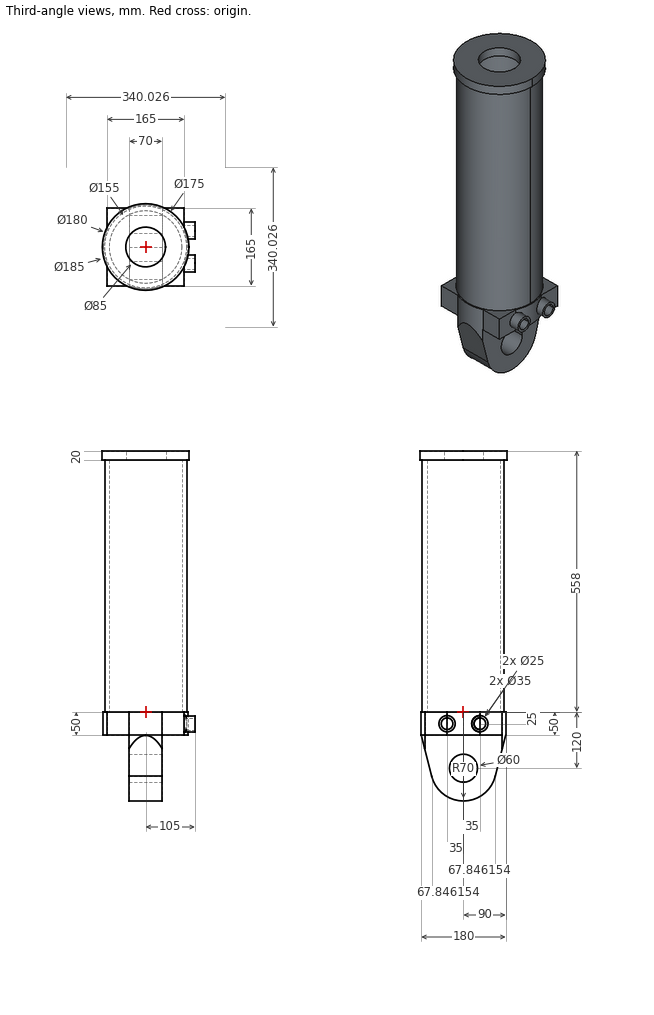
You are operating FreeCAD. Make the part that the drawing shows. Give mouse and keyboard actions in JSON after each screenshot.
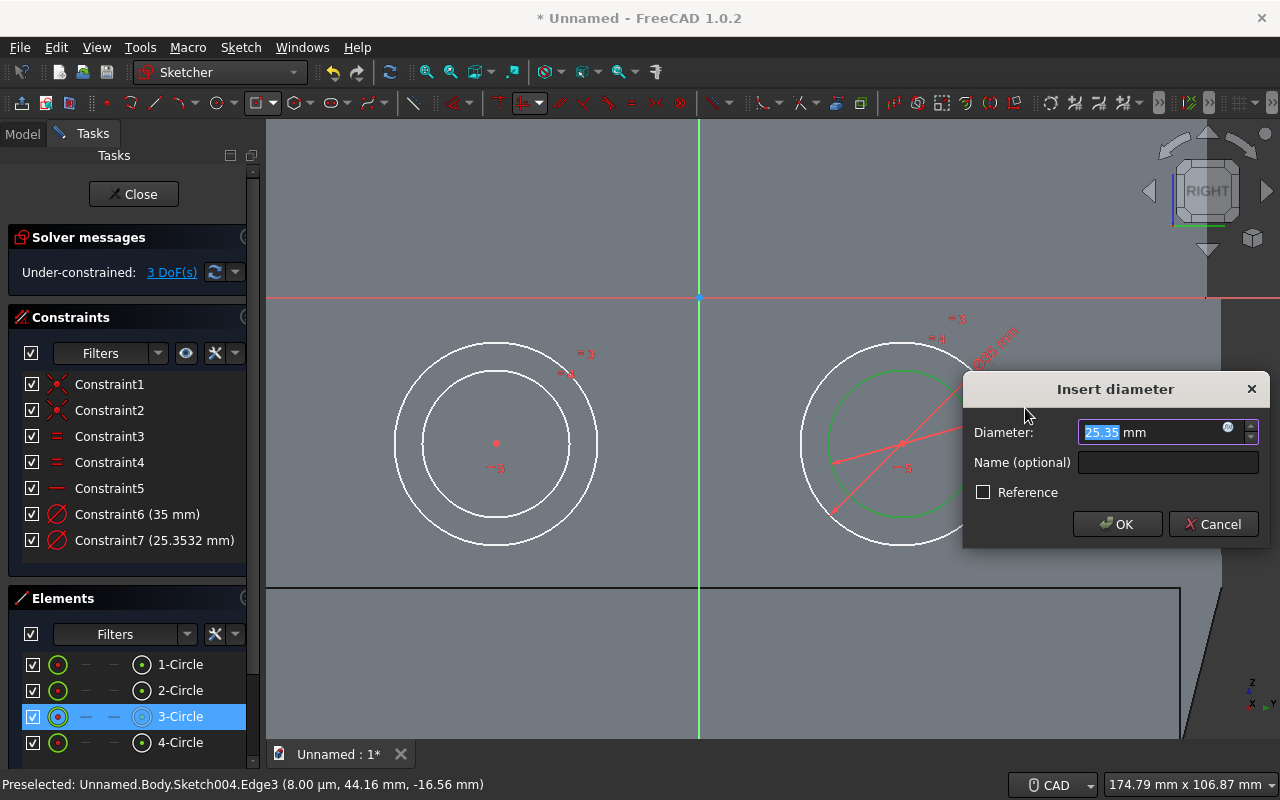
{"action": "type", "text": "25"}
{"action": "key", "text": "Return"}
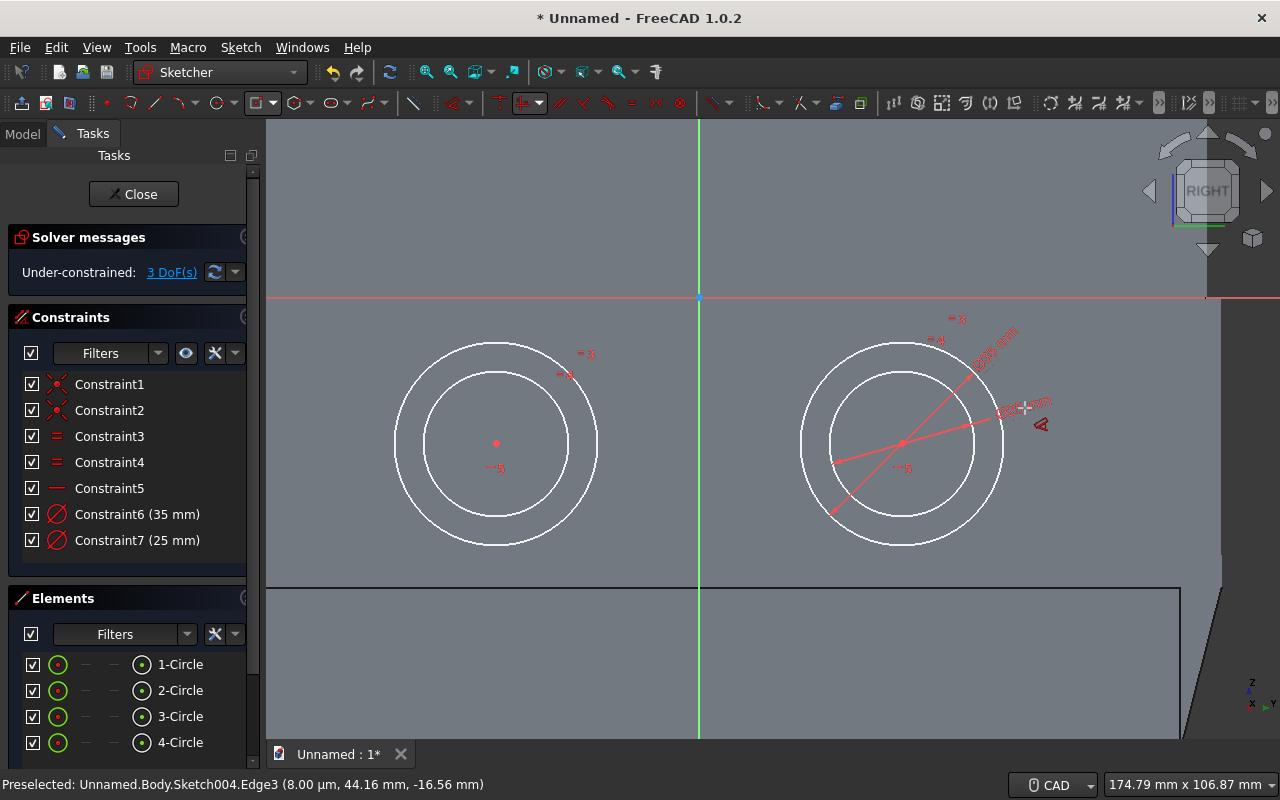
{"action": "left_click", "coordinate": [902, 444]}
{"action": "left_click", "coordinate": [801, 264]}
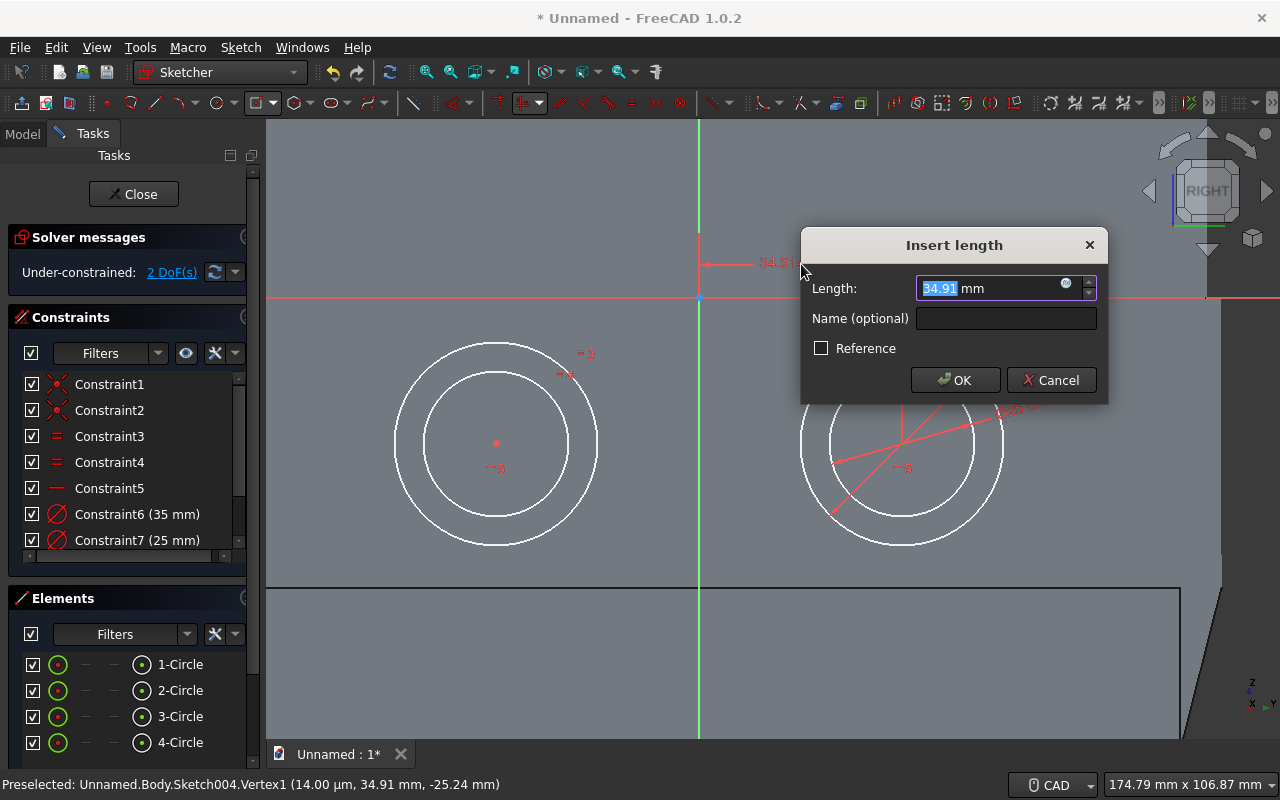
{"action": "type", "text": "35"}
{"action": "key", "text": "Return"}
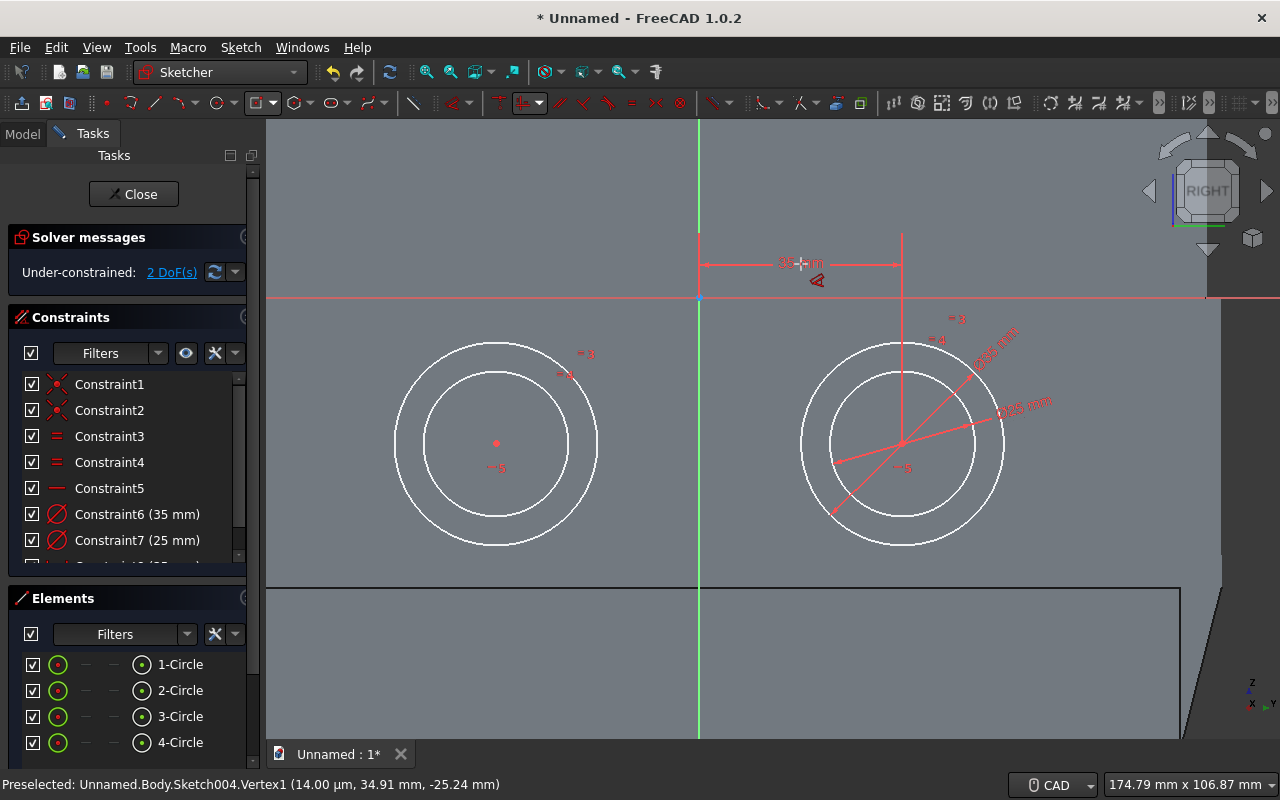
{"action": "left_click", "coordinate": [902, 444]}
{"action": "left_click", "coordinate": [936, 404]}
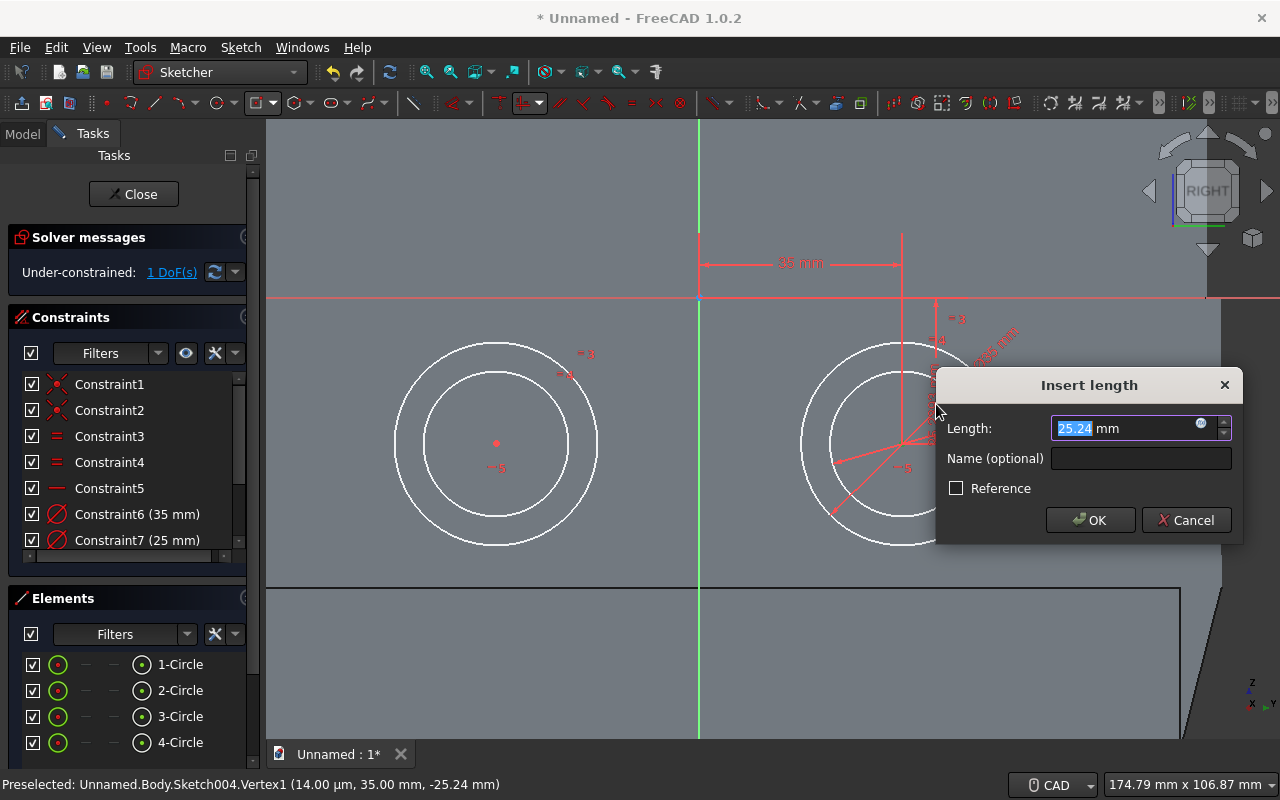
{"action": "type", "text": "25"}
{"action": "key", "text": "Return"}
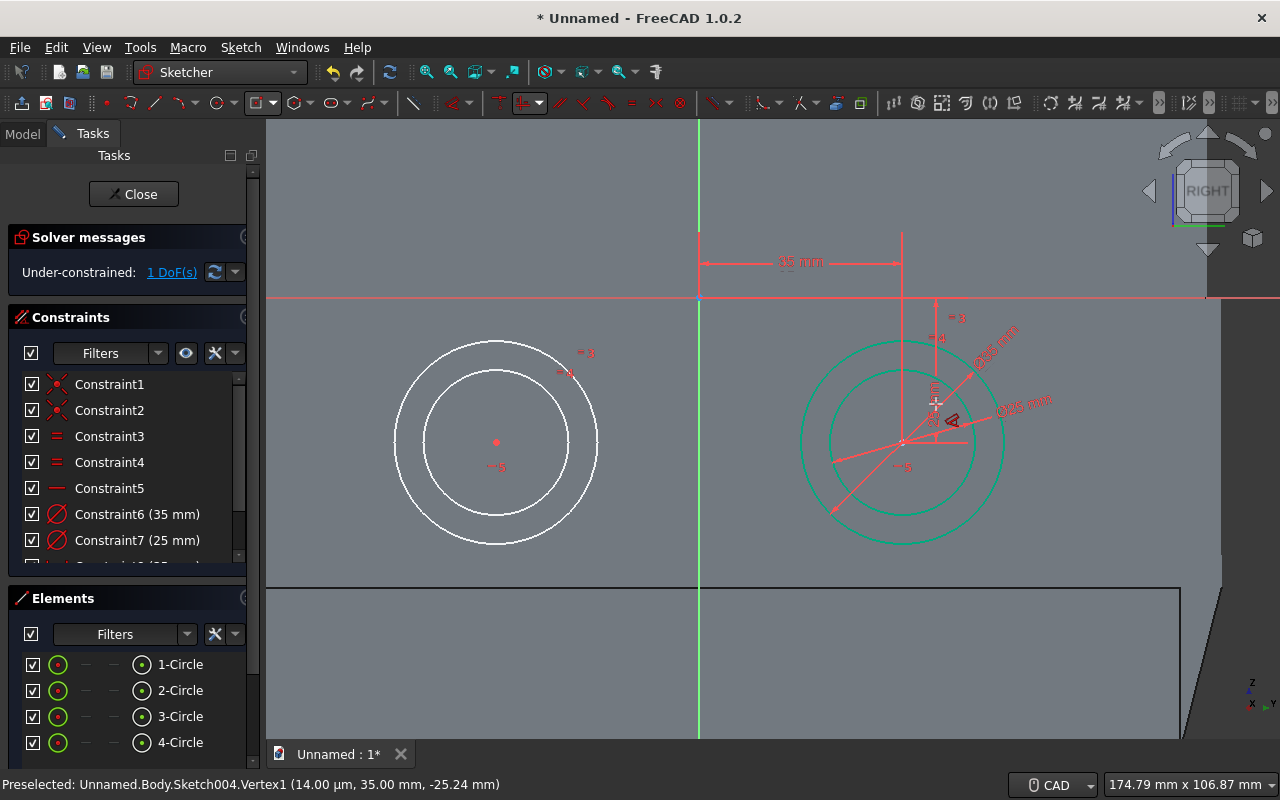
{"action": "left_click", "coordinate": [496, 443]}
{"action": "left_click", "coordinate": [598, 264]}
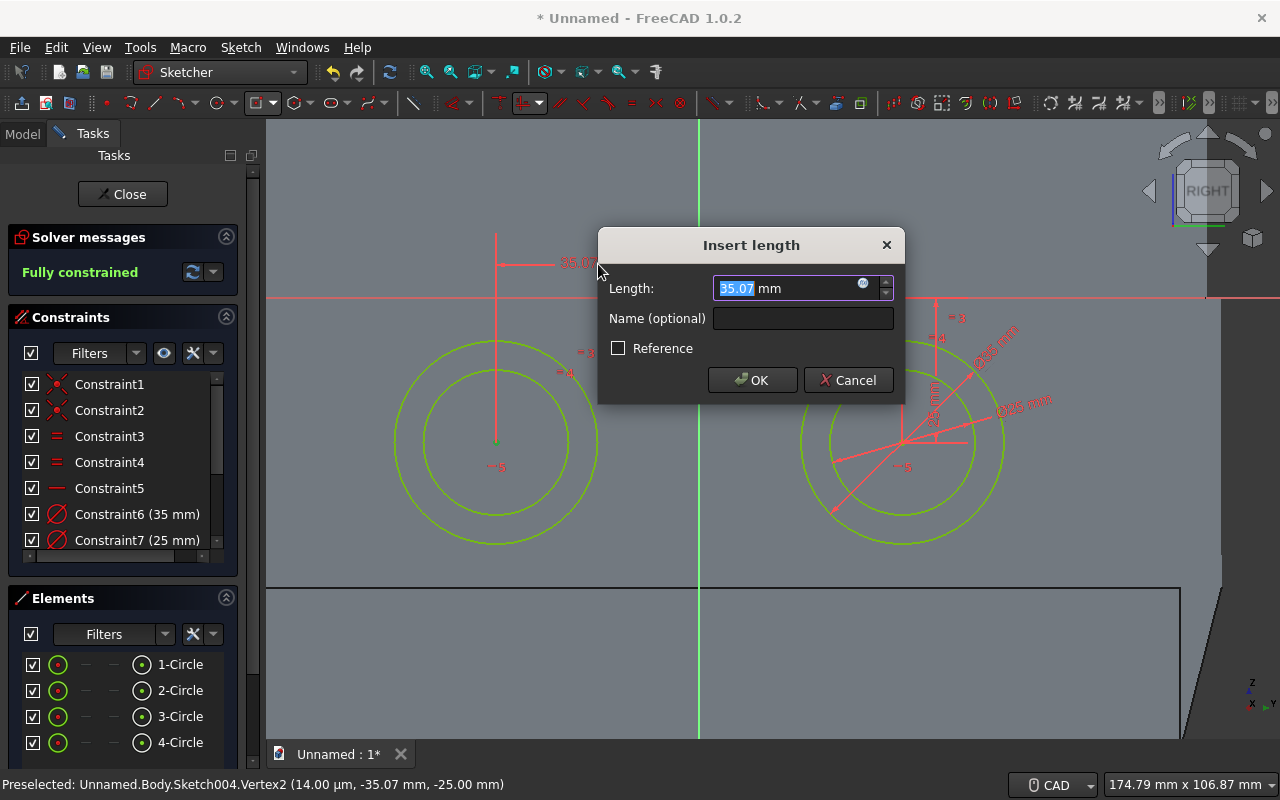
{"action": "type", "text": "35"}
{"action": "key", "text": "Return"}
{"action": "key", "text": "Escape"}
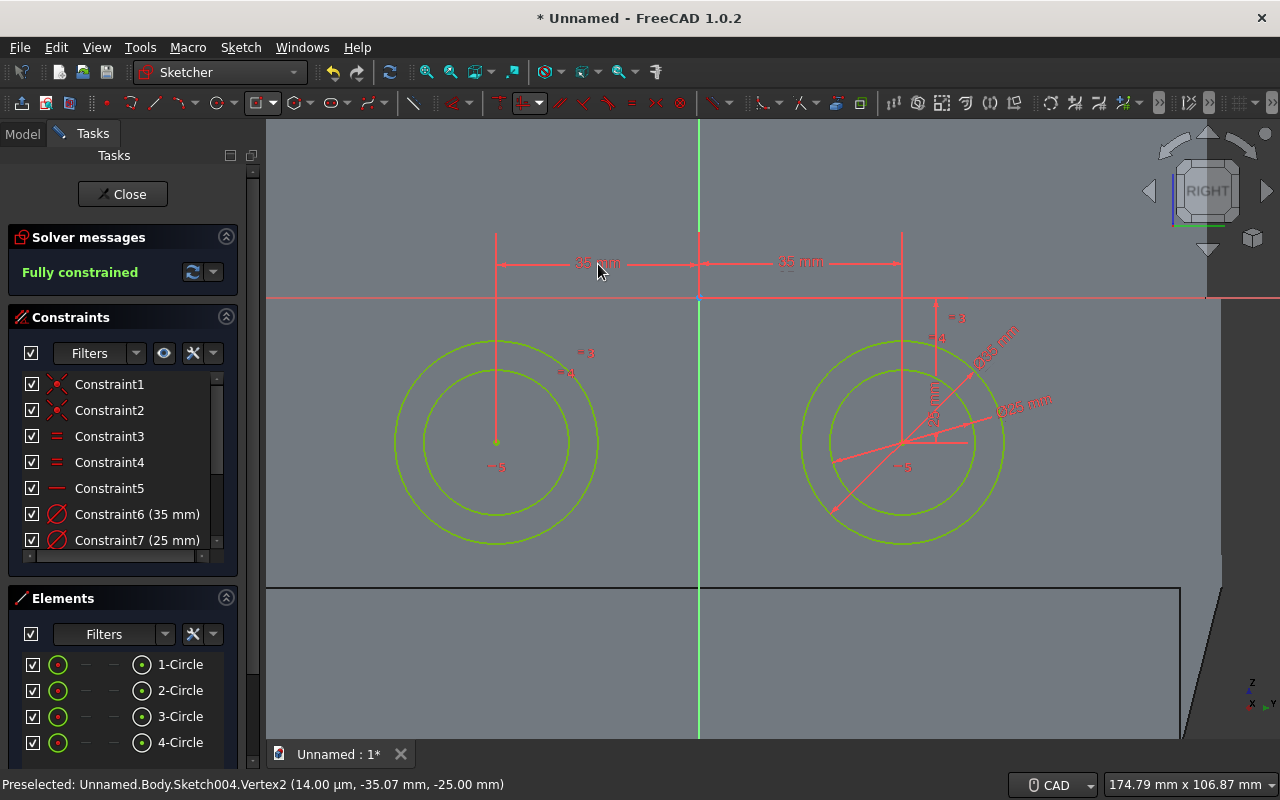
{"action": "left_click", "coordinate": [123, 194]}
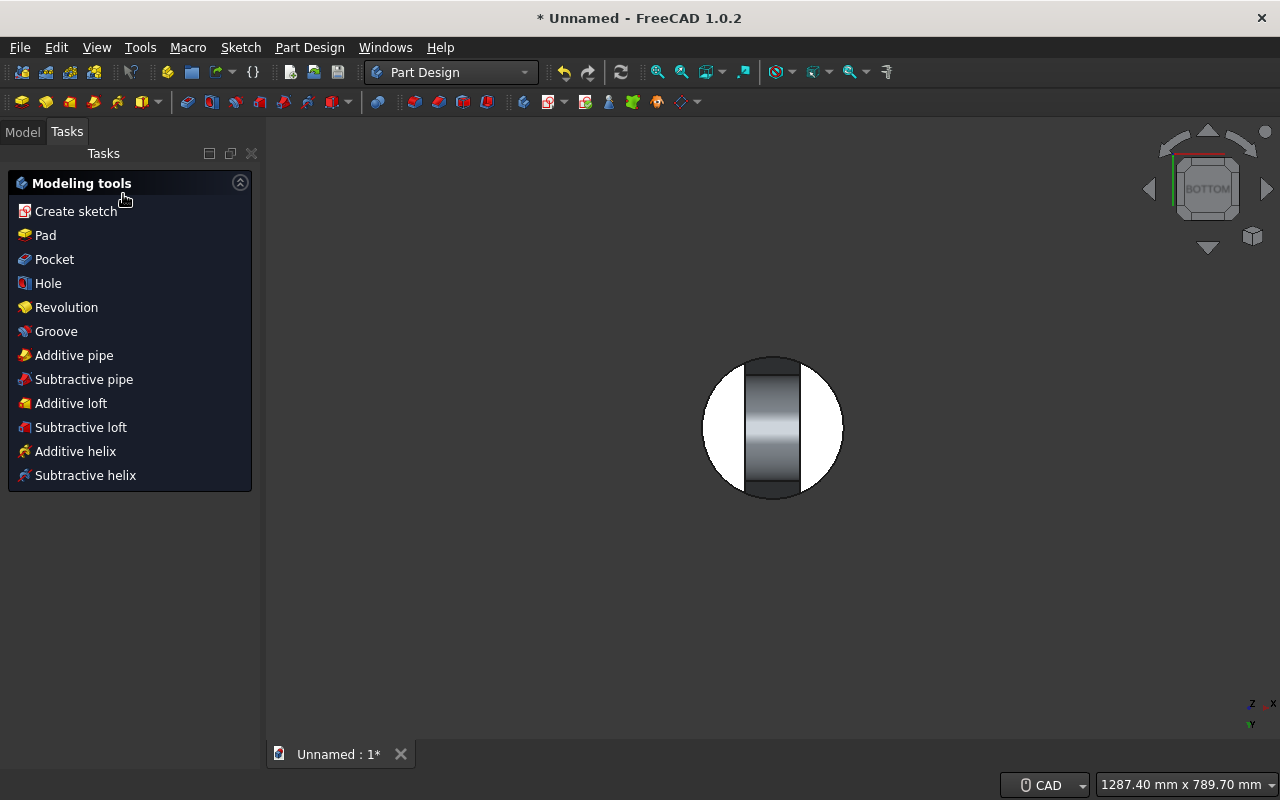
{"action": "left_click", "coordinate": [22, 102]}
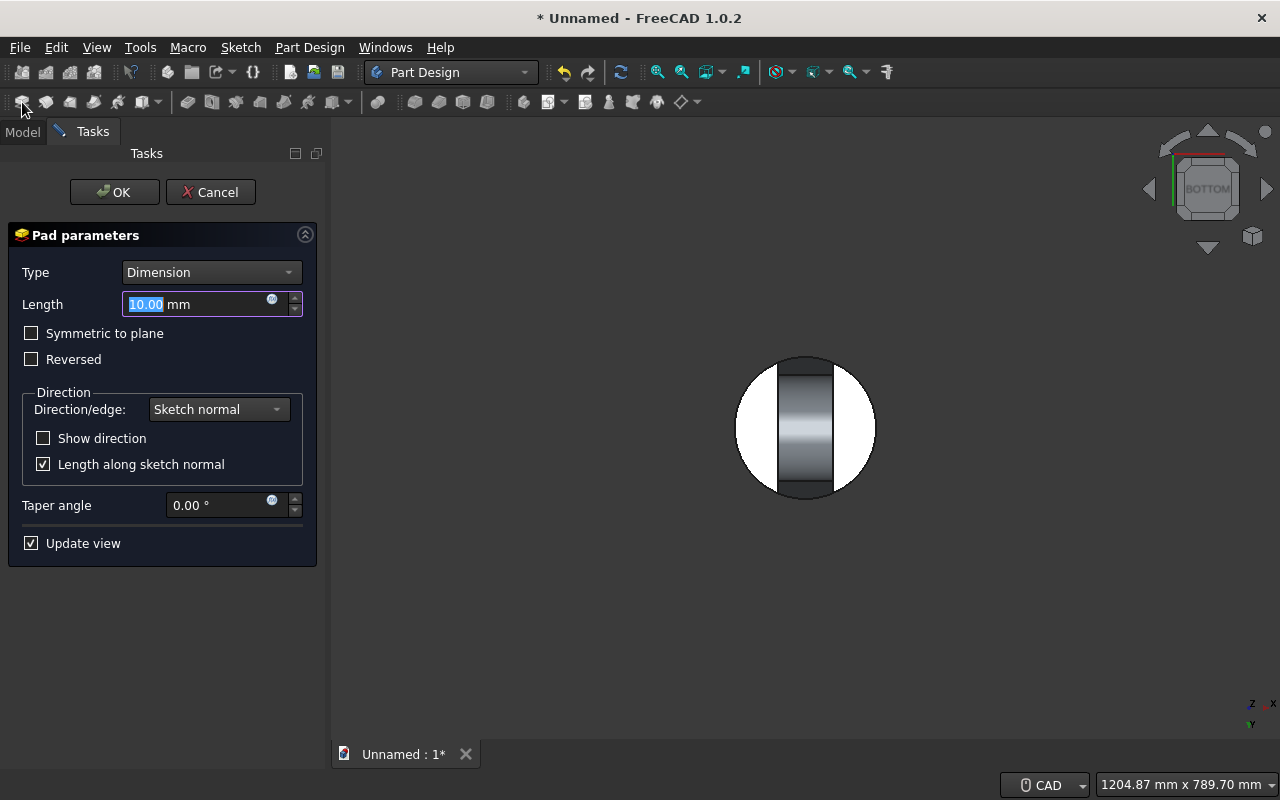
{"action": "type", "text": "105"}
{"action": "key", "text": "Tab"}